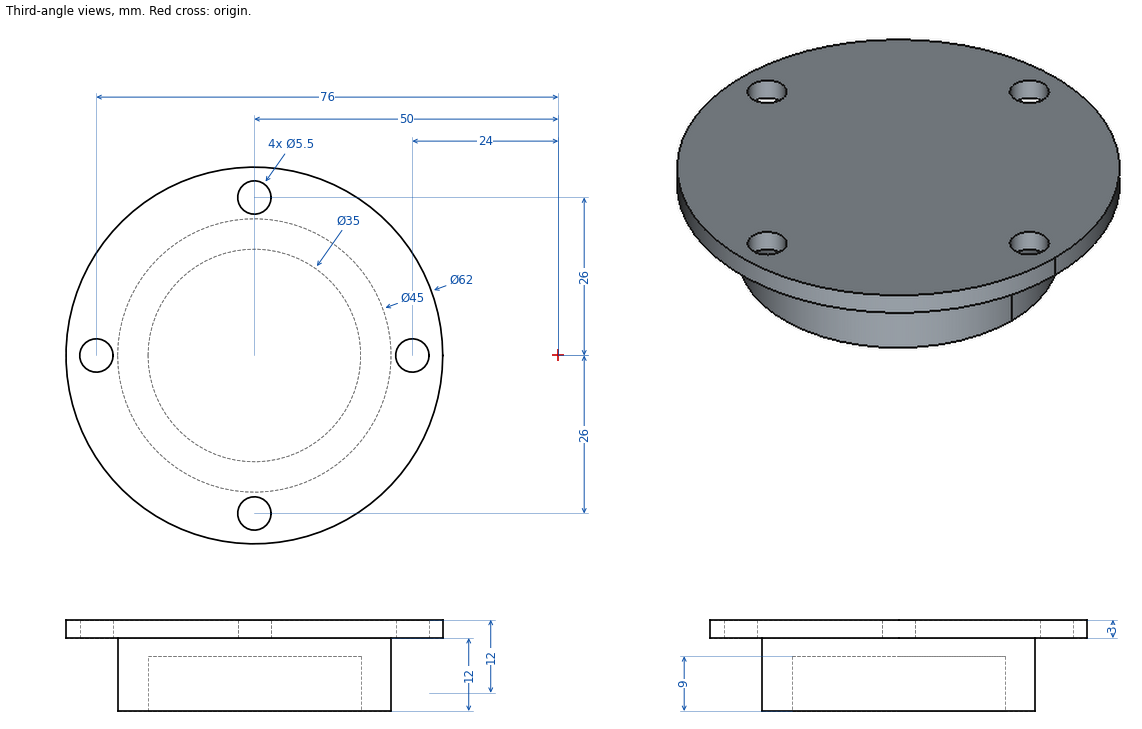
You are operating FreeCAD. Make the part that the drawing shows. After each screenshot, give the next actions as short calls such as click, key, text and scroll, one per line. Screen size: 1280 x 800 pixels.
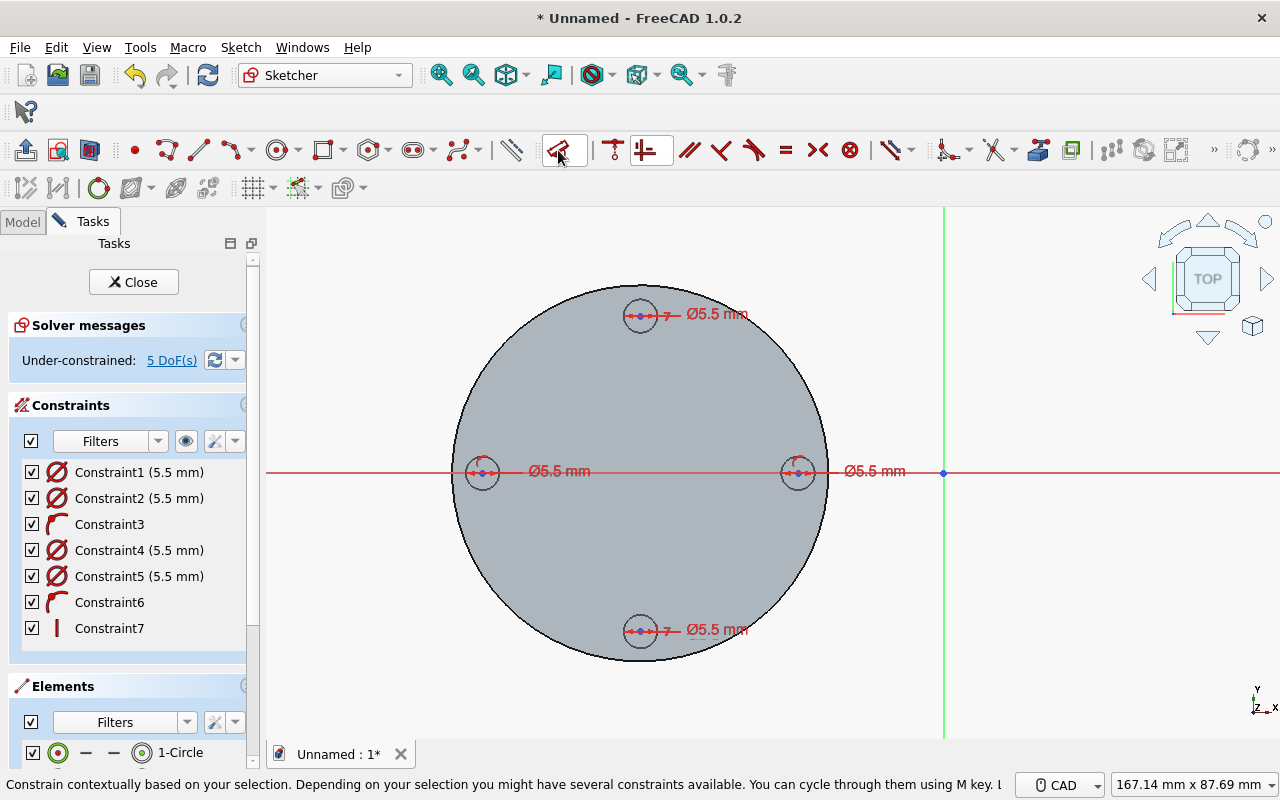
click(641, 316)
click(792, 282)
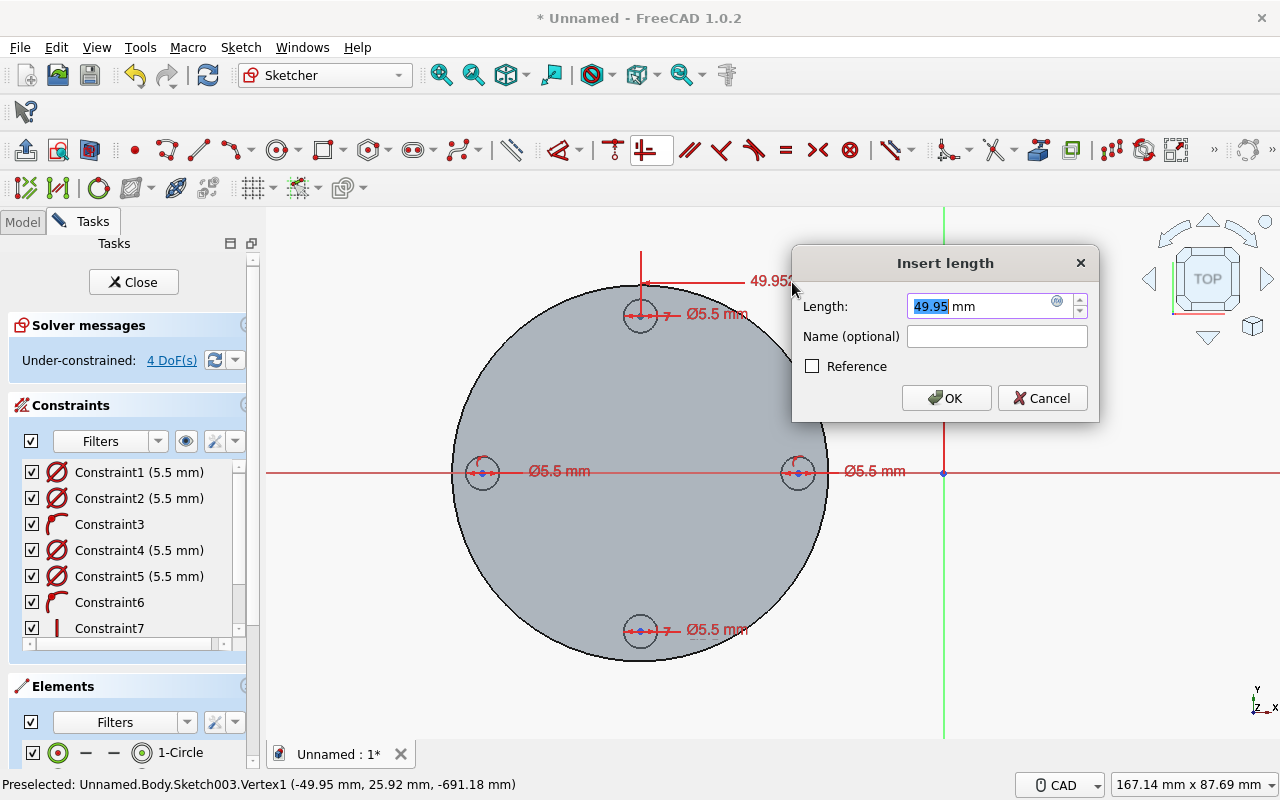
text(50)
key(Return)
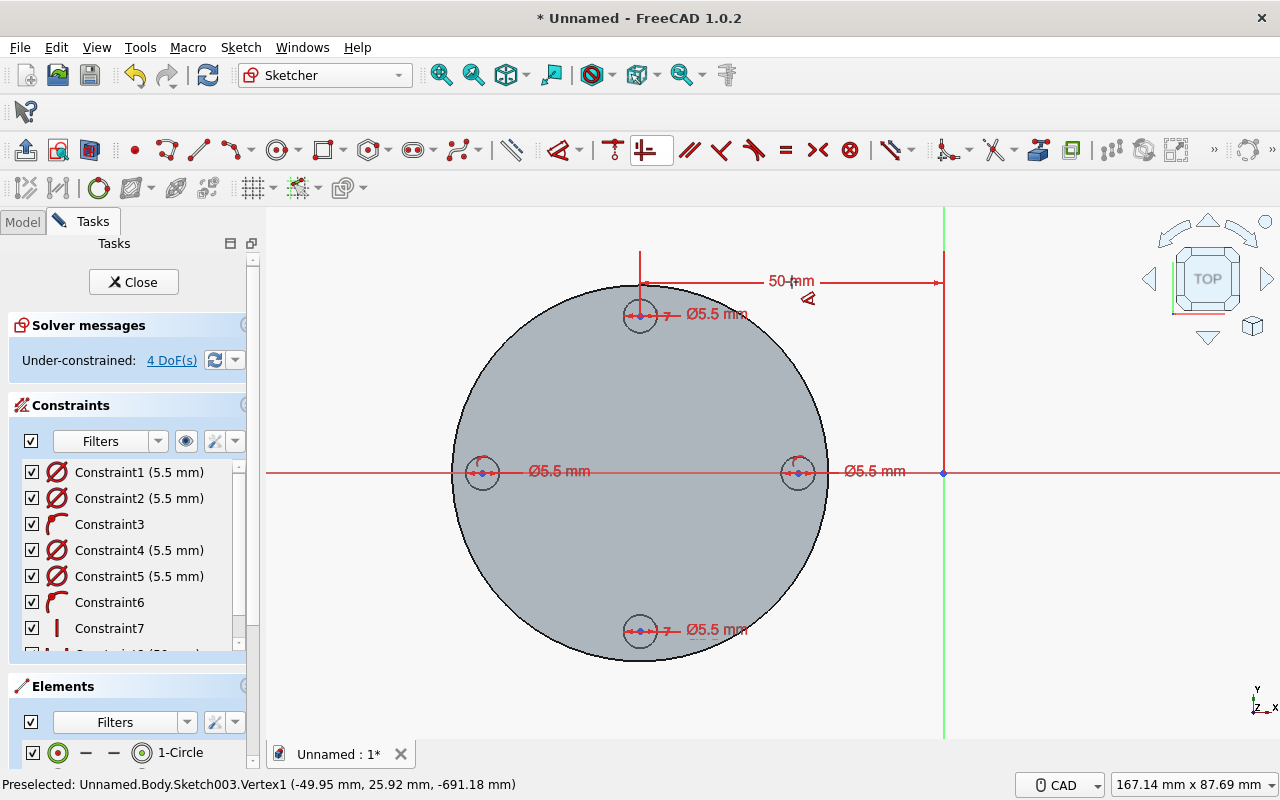
click(640, 316)
click(978, 395)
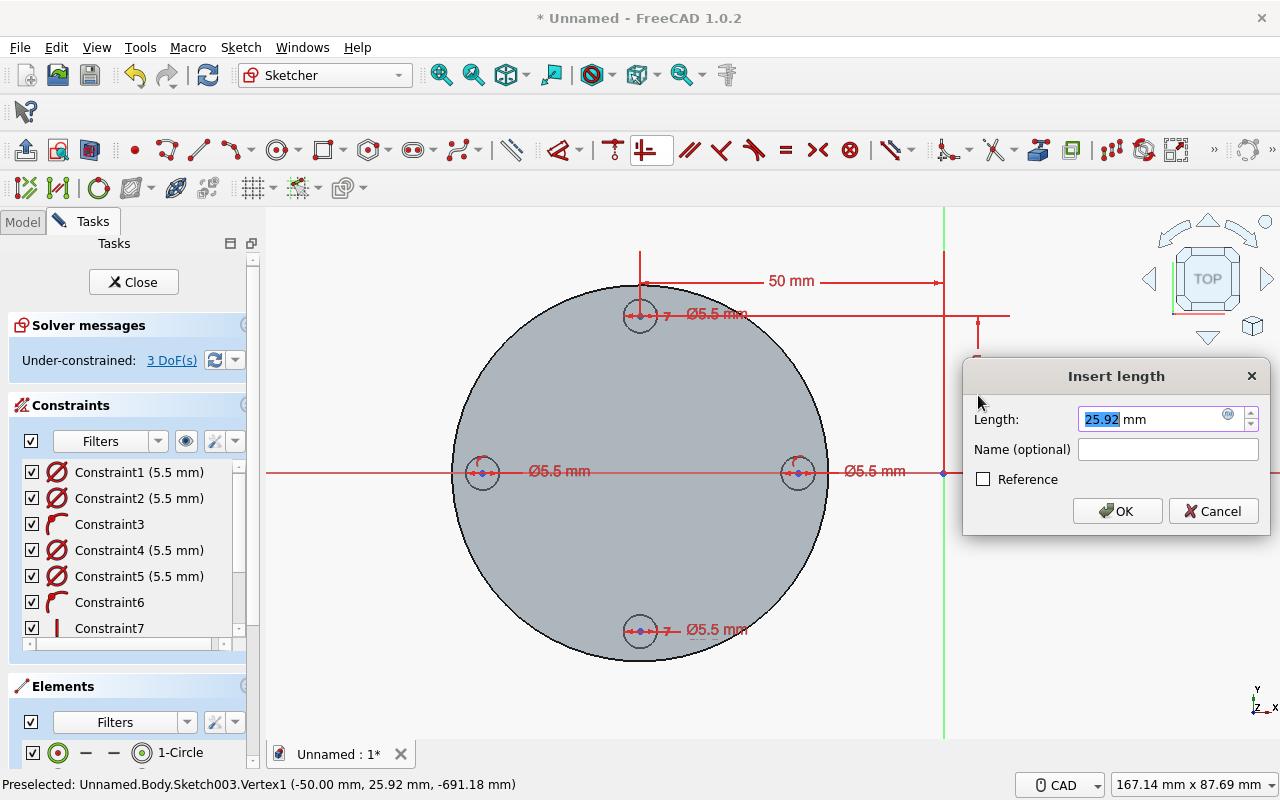
text(26)
key(Return)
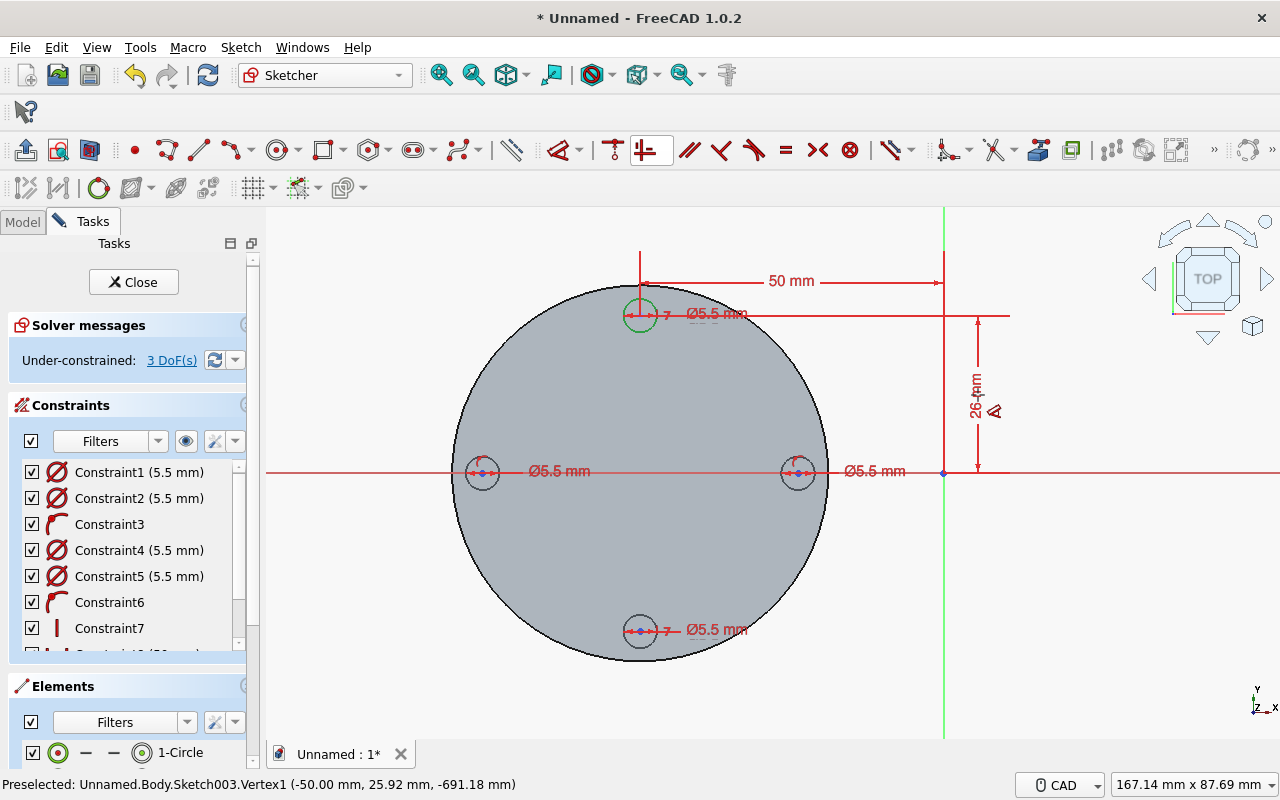
click(798, 473)
click(871, 507)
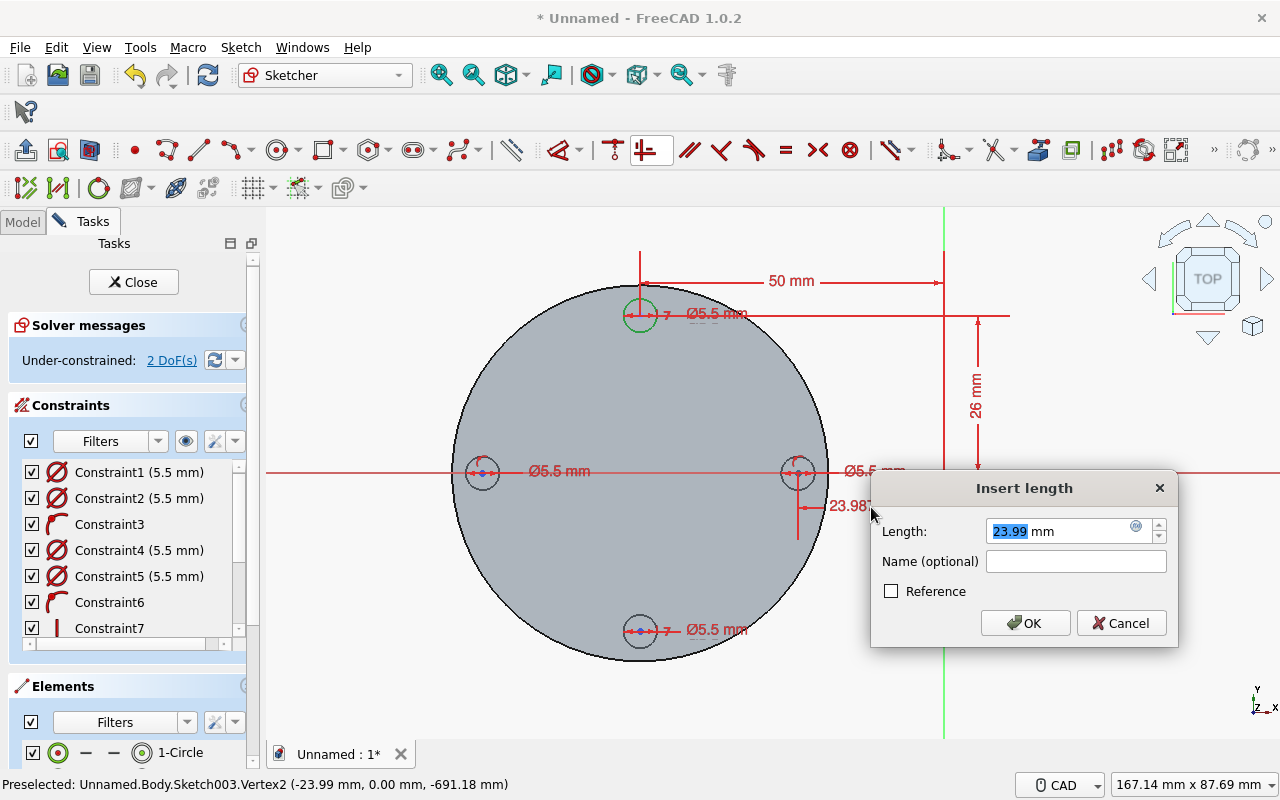
text(24)
key(Return)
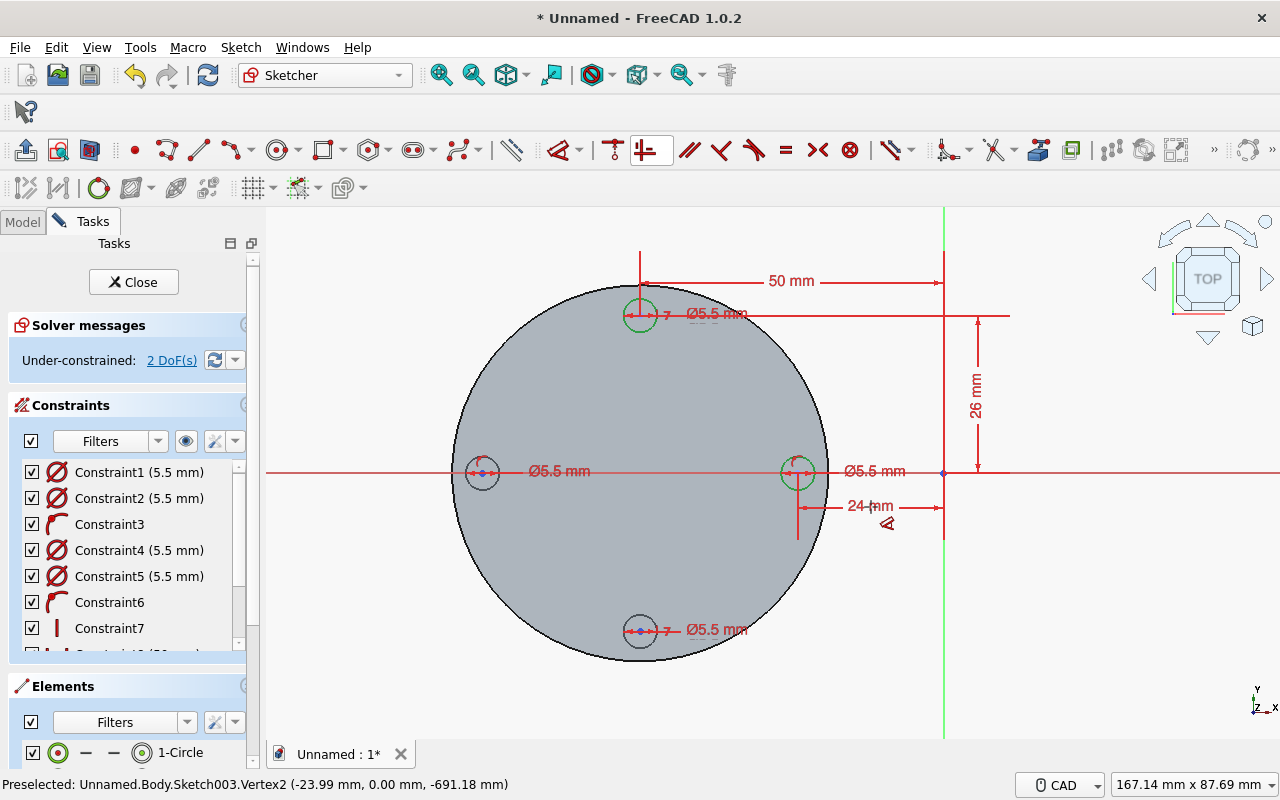
click(640, 632)
click(978, 552)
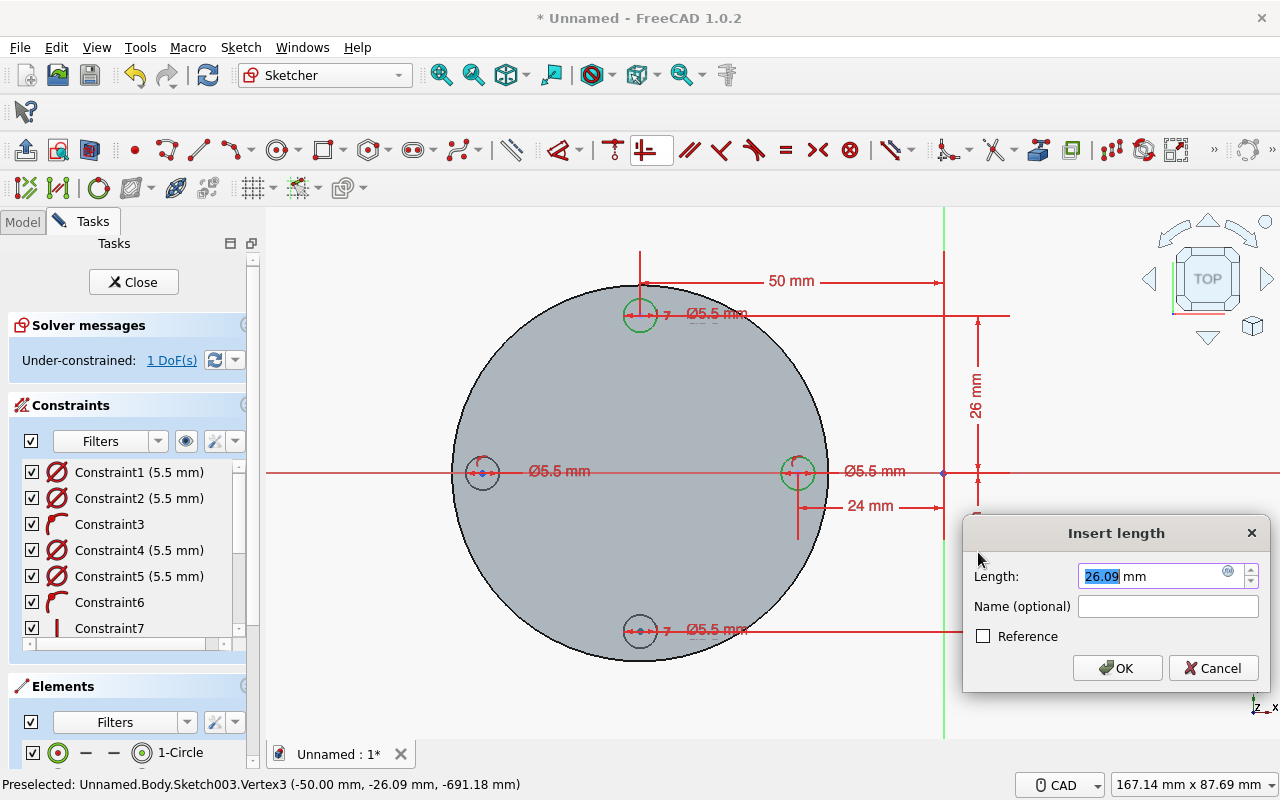
text(26)
key(Return)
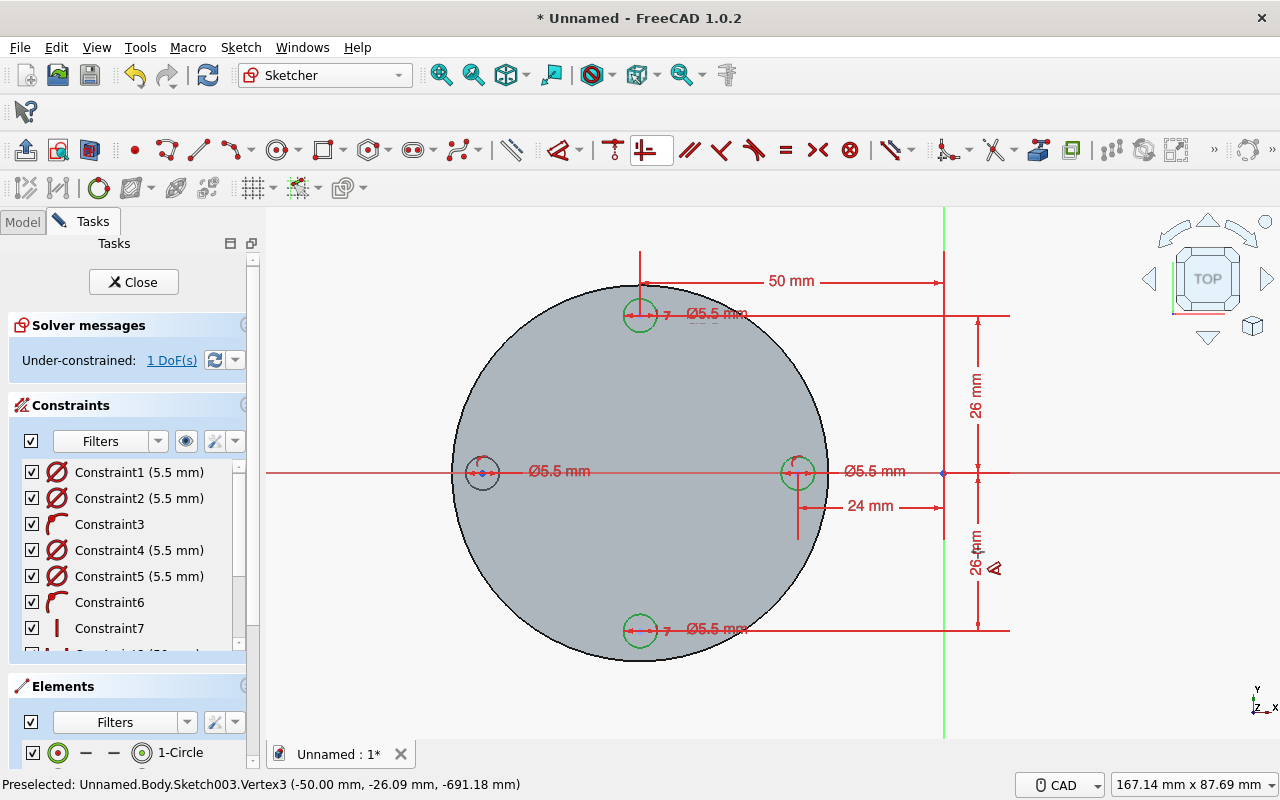
click(483, 473)
click(713, 507)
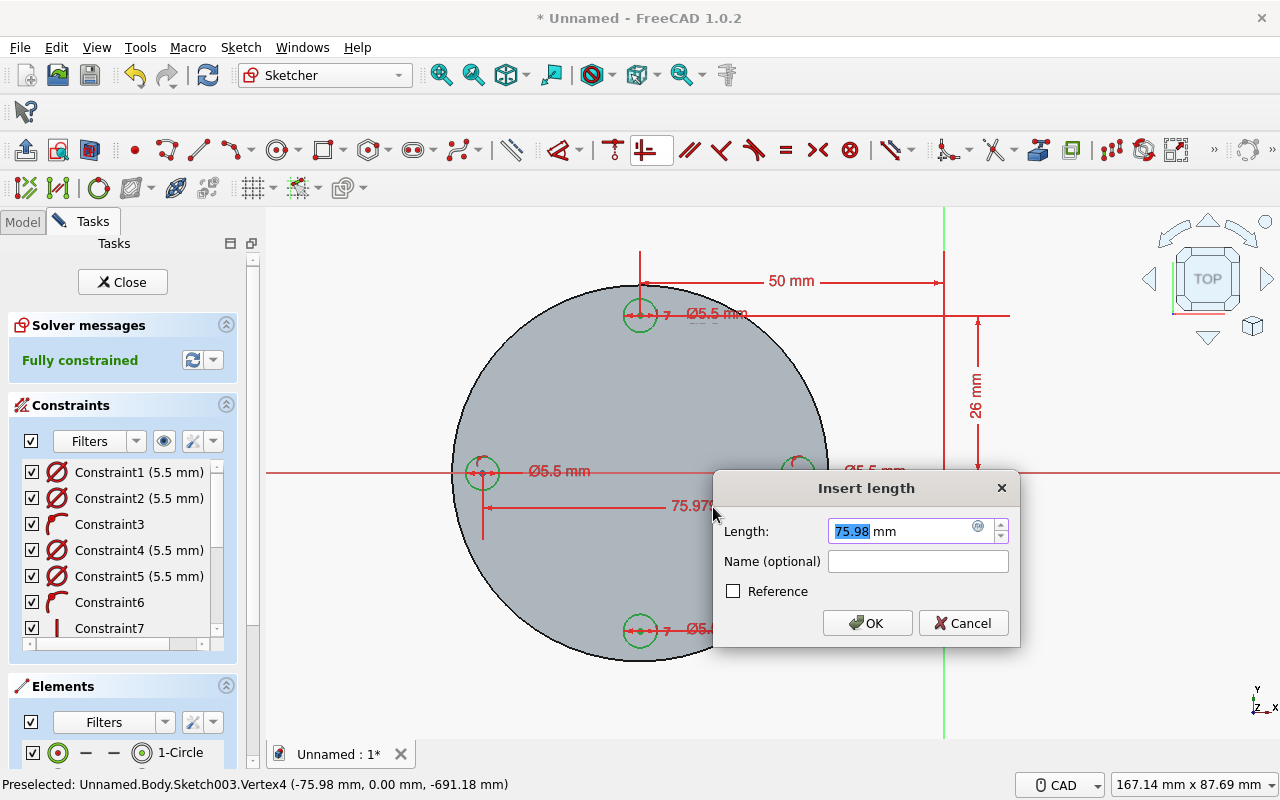
text(76)
key(Return)
key(Escape)